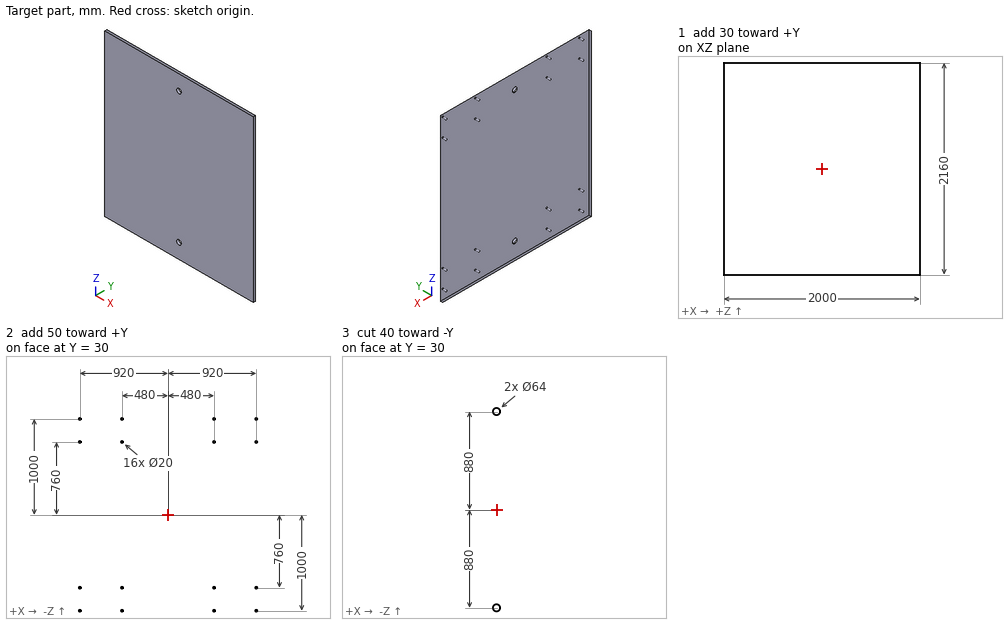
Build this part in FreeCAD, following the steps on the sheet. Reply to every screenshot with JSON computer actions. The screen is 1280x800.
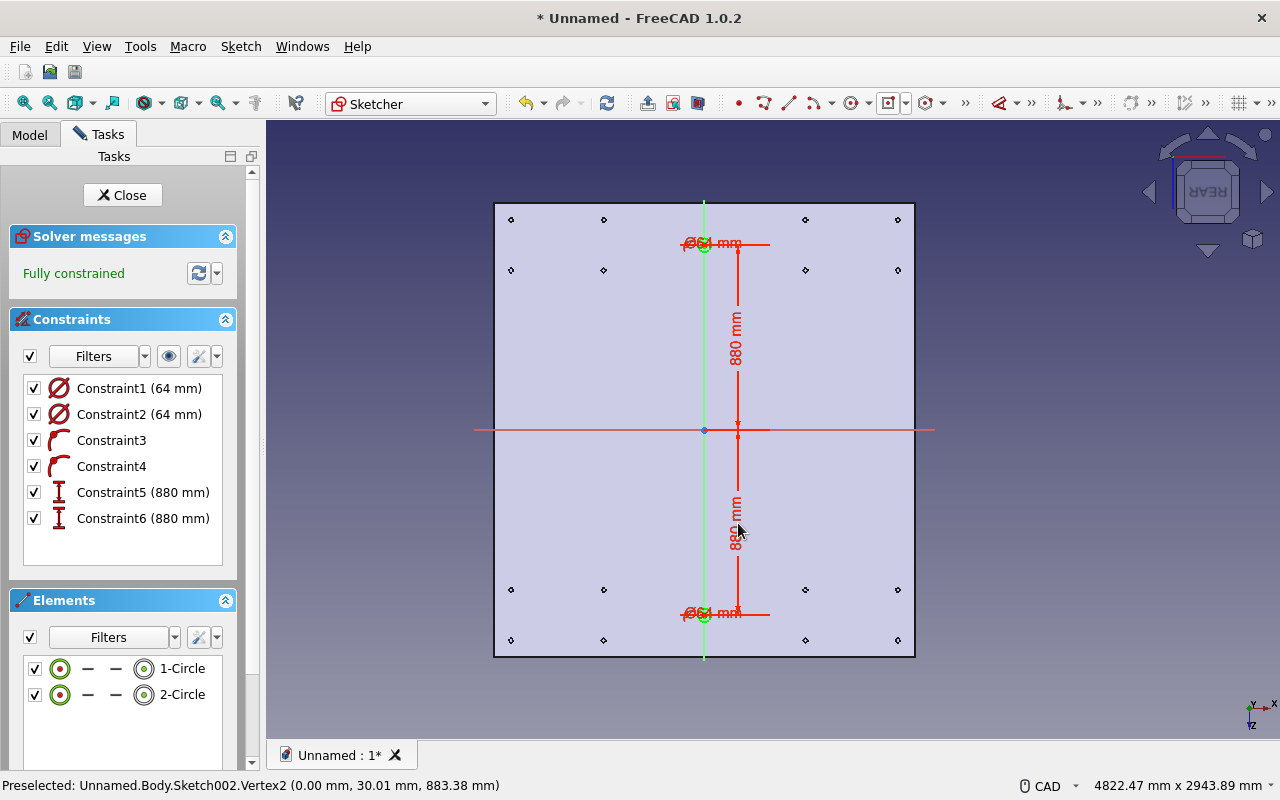
{"action": "left_click", "coordinate": [123, 195]}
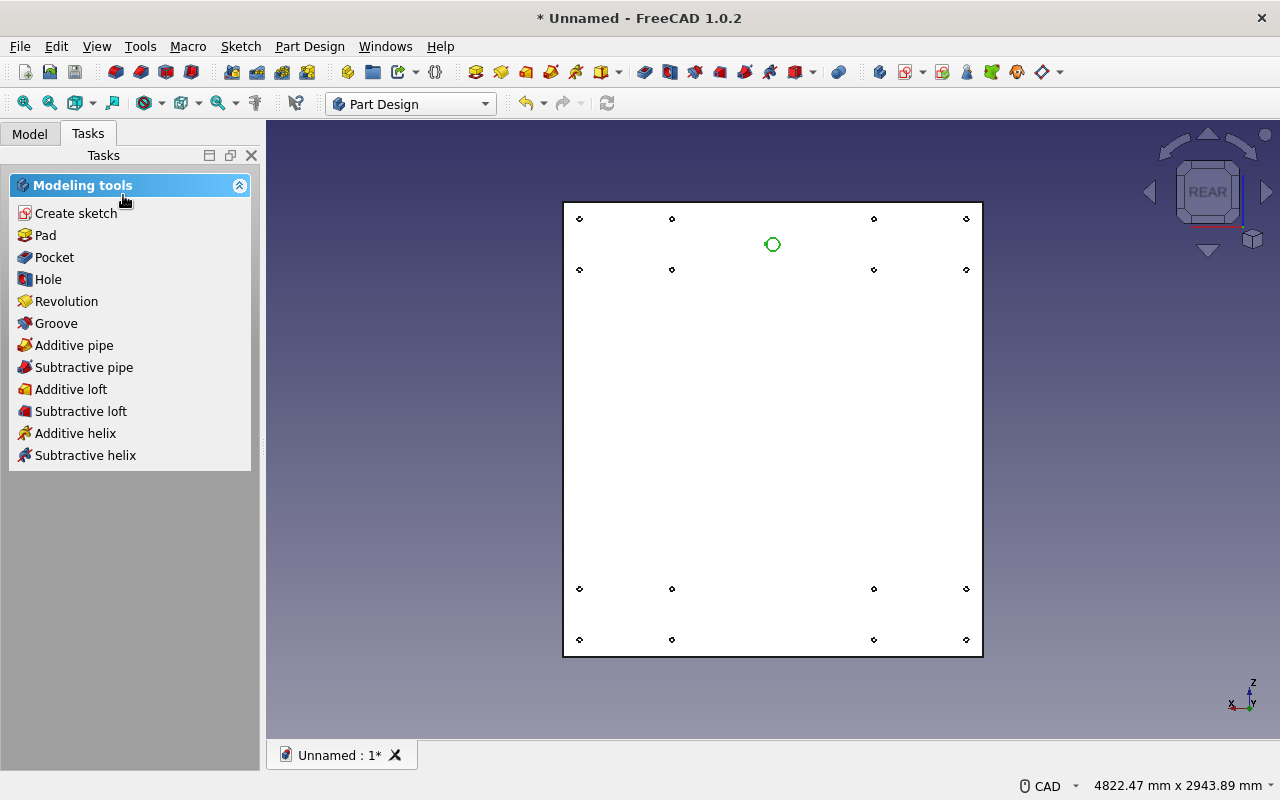
{"action": "left_click", "coordinate": [645, 72]}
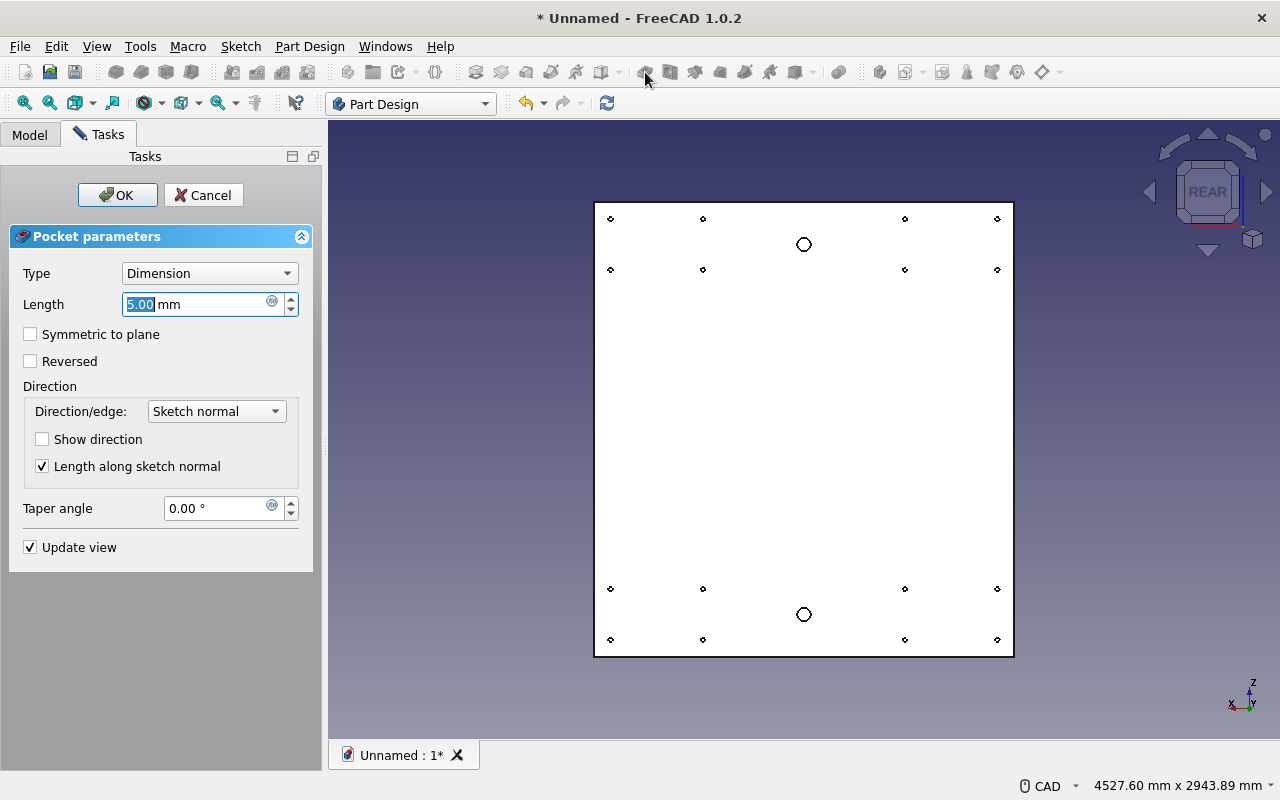
{"action": "type", "text": "40"}
{"action": "key", "text": "Tab"}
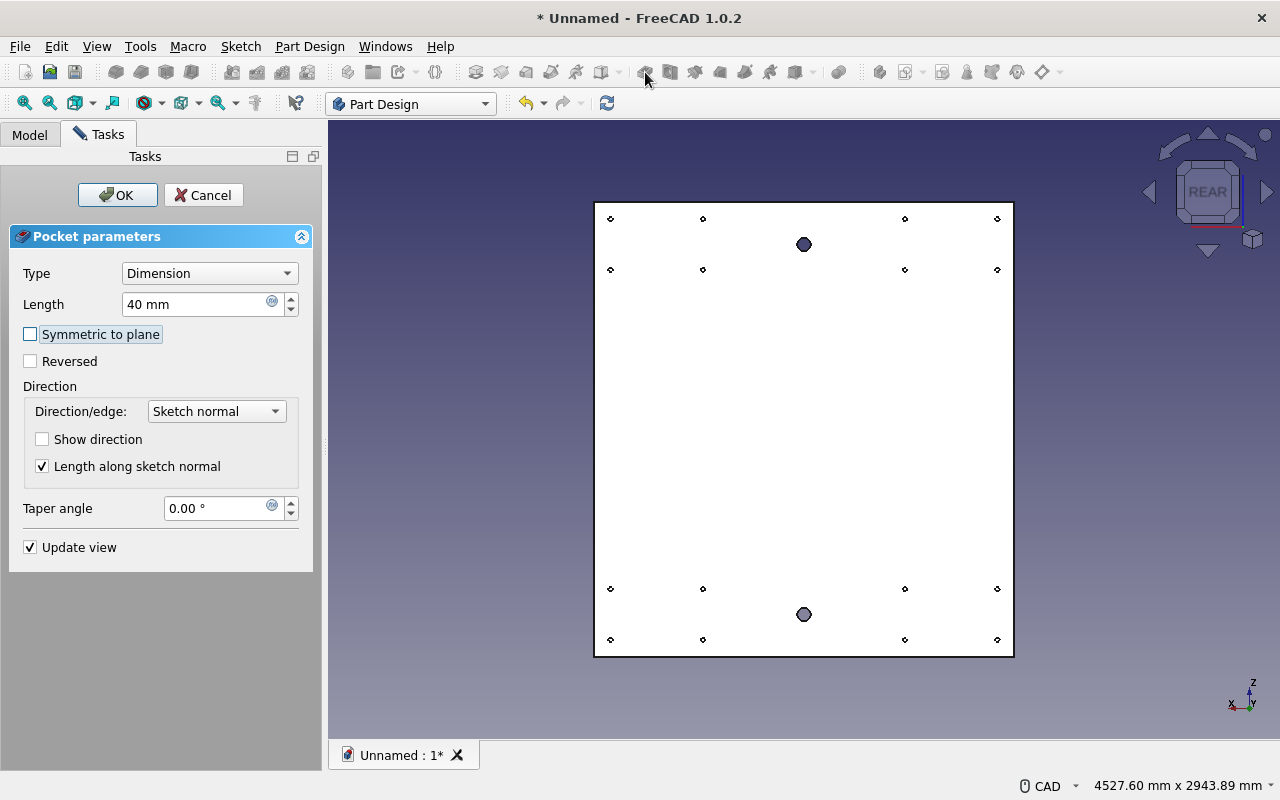
{"action": "left_click", "coordinate": [118, 195]}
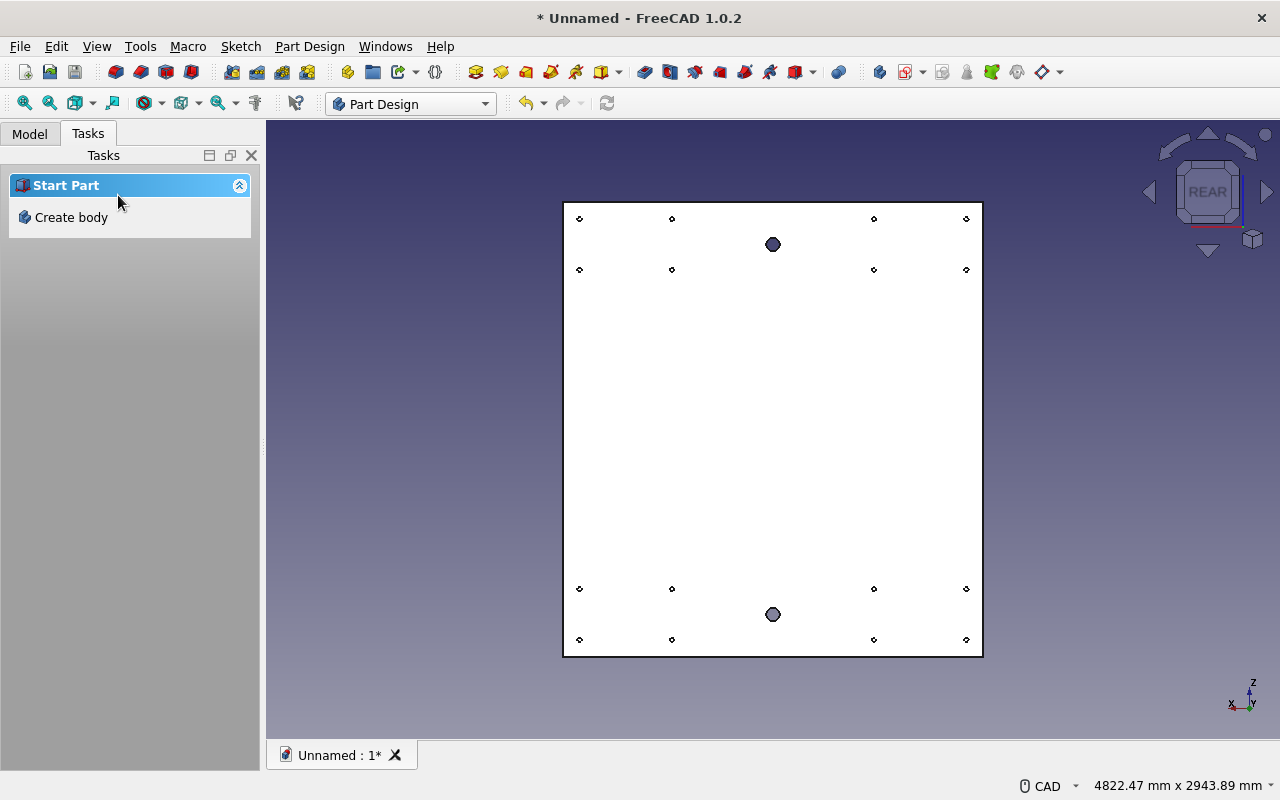
{"action": "key", "text": "0"}